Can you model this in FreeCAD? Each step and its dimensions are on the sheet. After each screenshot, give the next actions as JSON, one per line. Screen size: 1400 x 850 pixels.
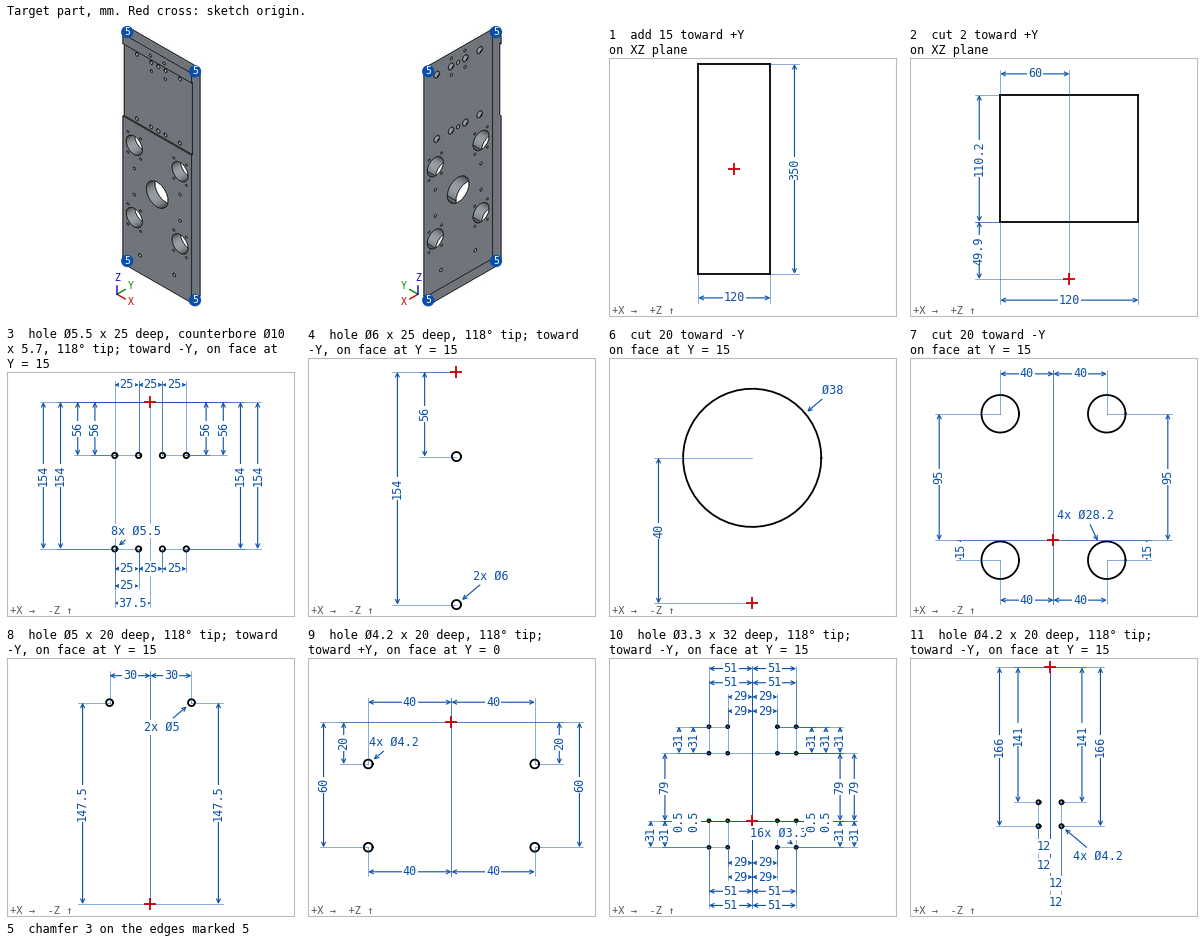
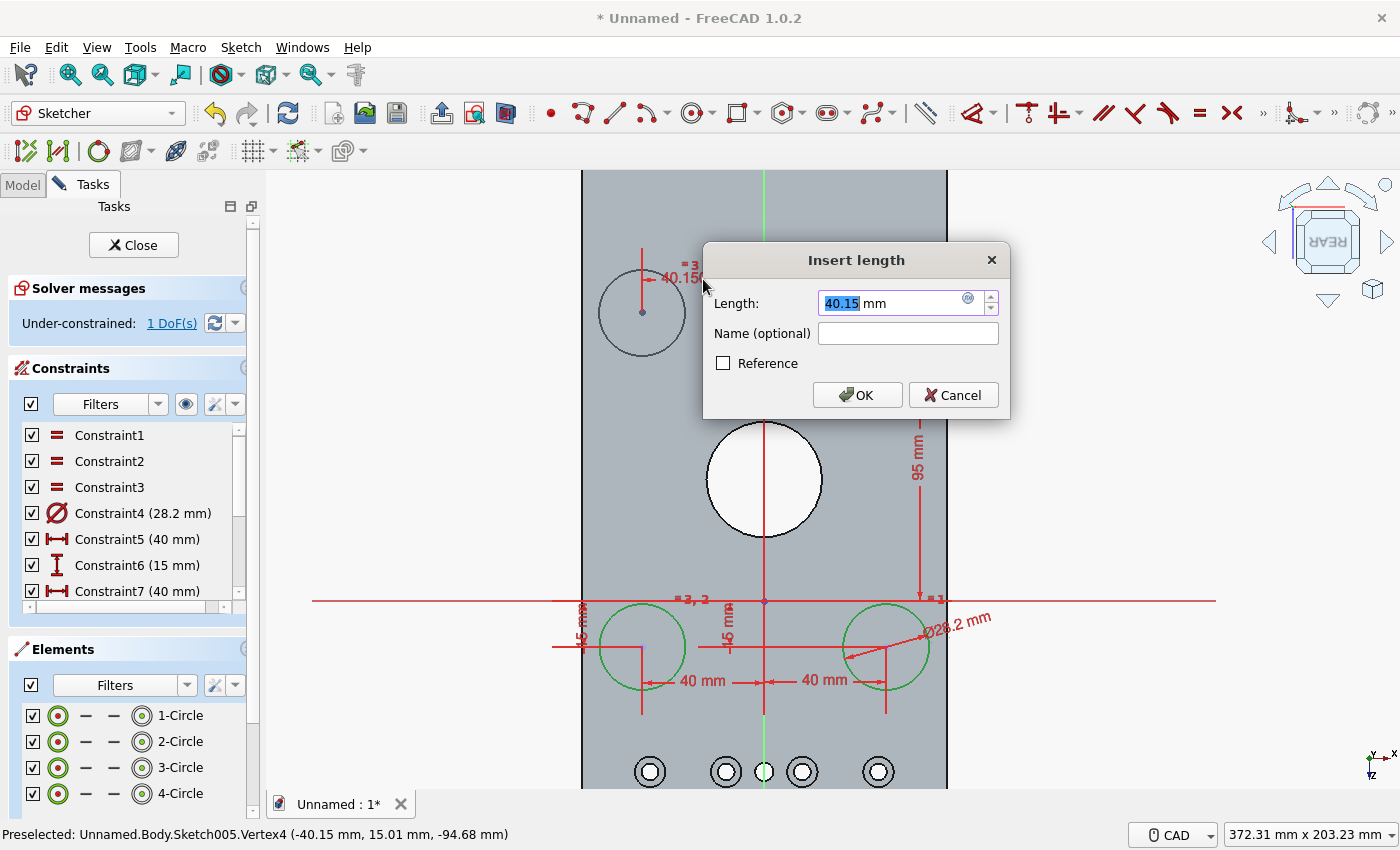
{"action": "type", "text": "40"}
{"action": "key", "text": "Return"}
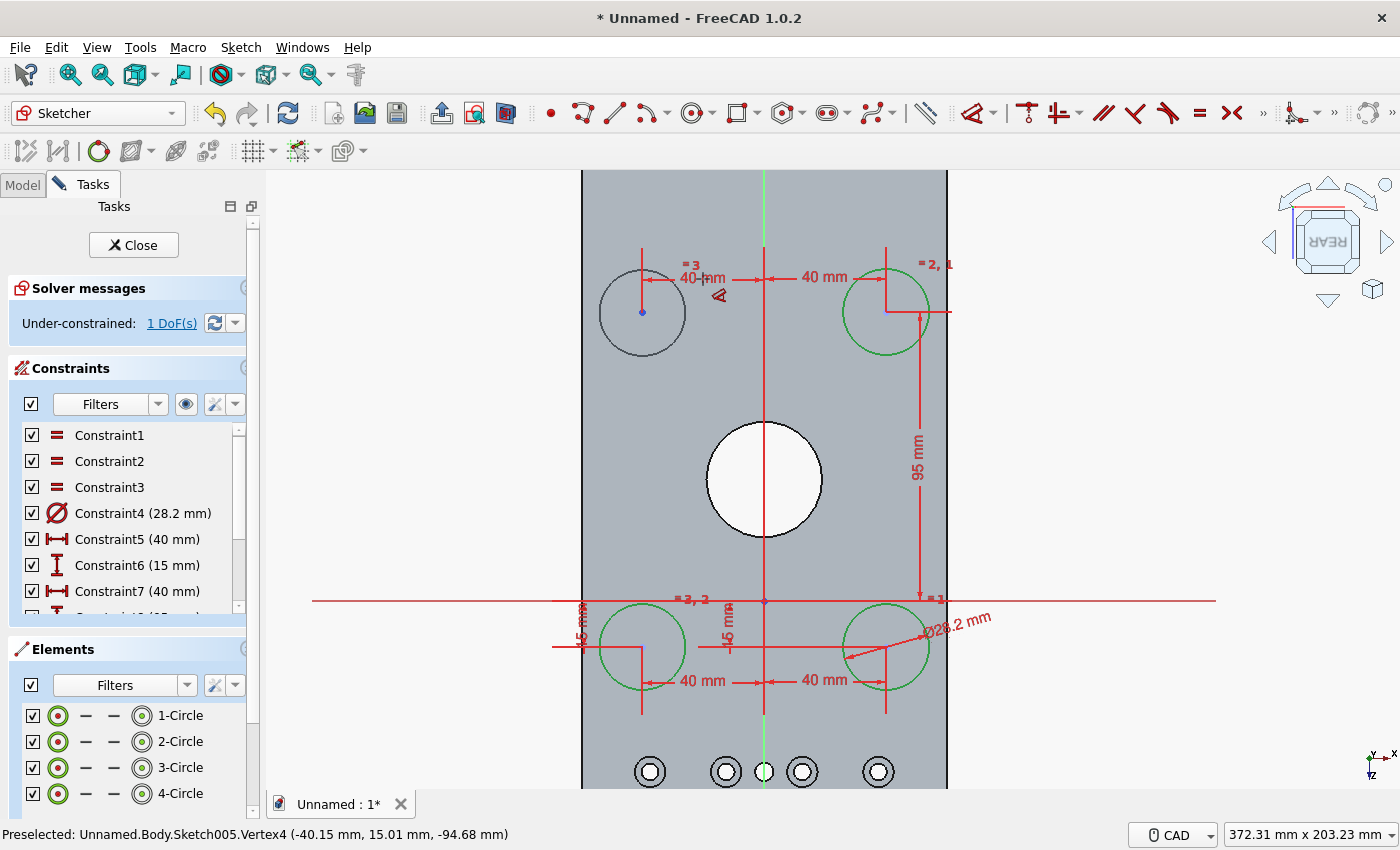
{"action": "left_click", "coordinate": [642, 313]}
{"action": "left_click", "coordinate": [608, 457]}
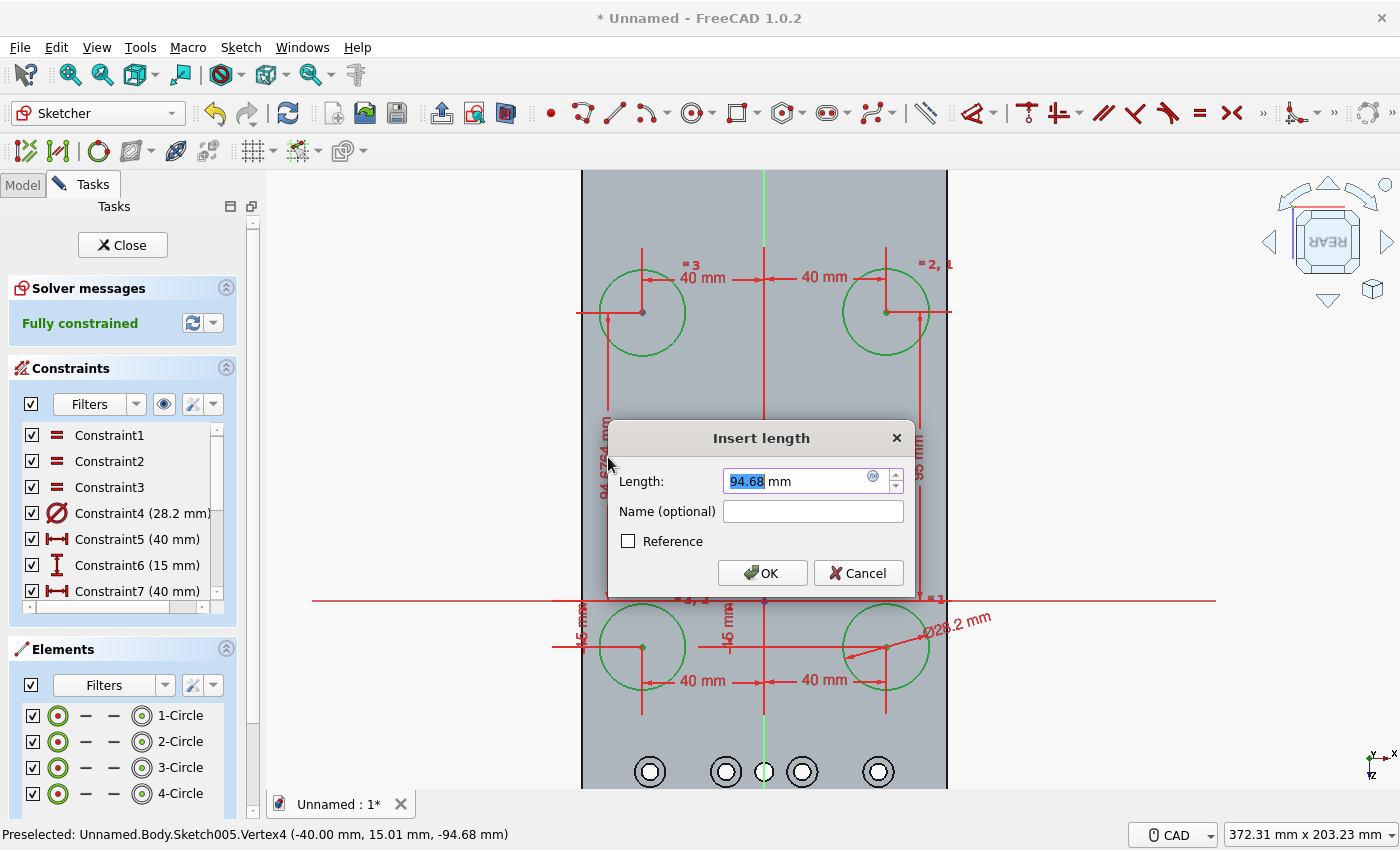
{"action": "type", "text": "95"}
{"action": "key", "text": "Return"}
{"action": "key", "text": "Escape"}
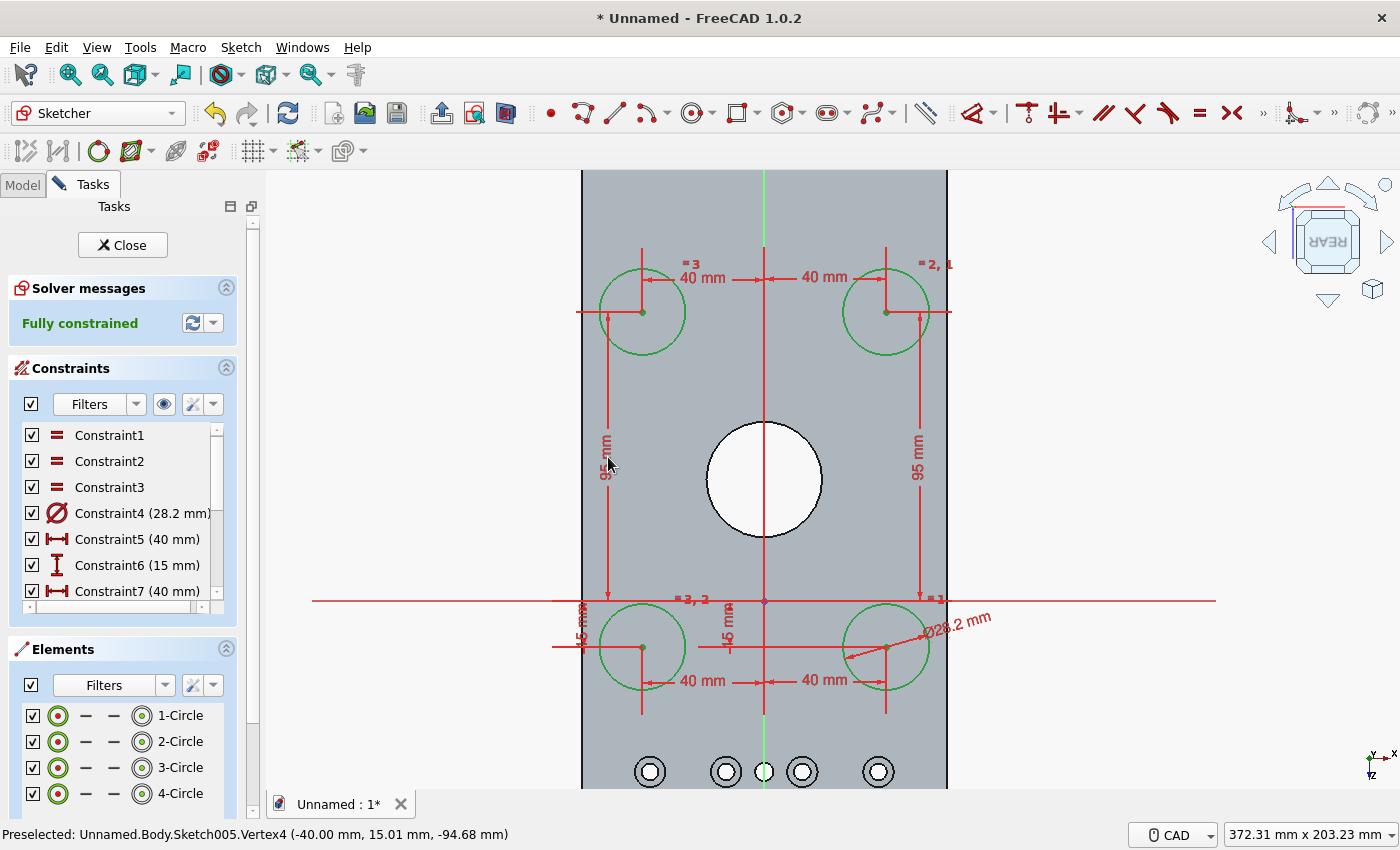
{"action": "left_click", "coordinate": [123, 245]}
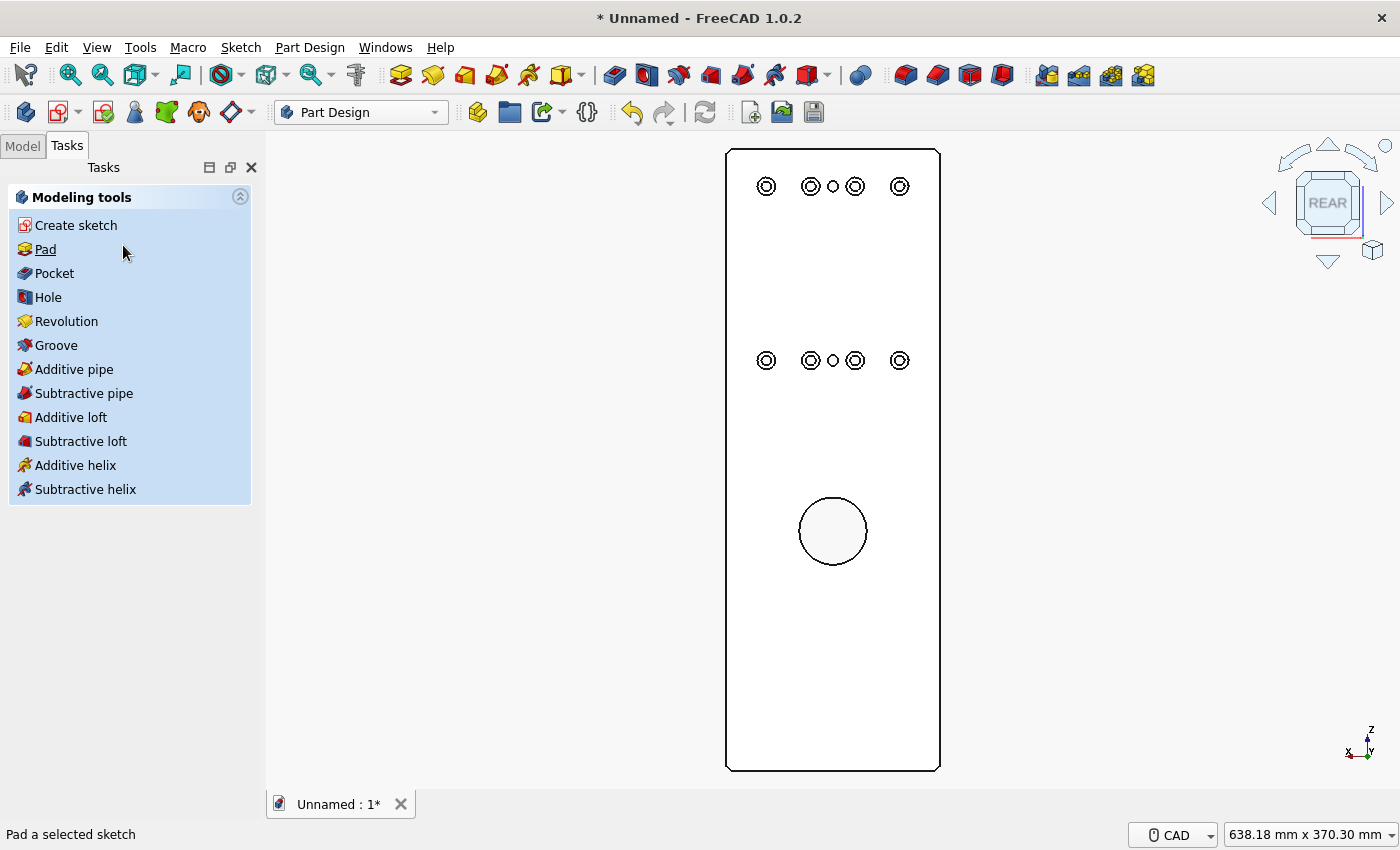
{"action": "left_click", "coordinate": [616, 76]}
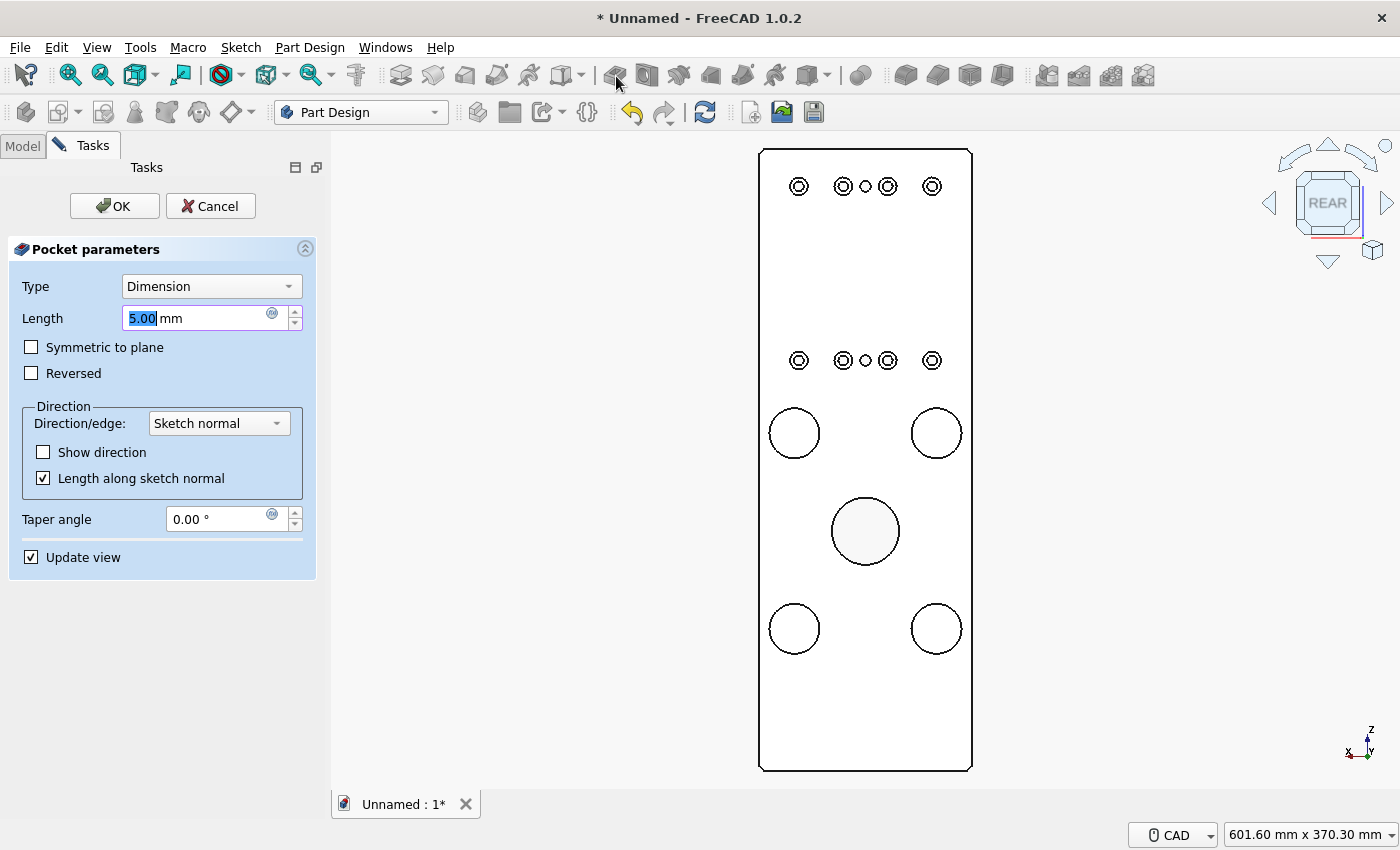
{"action": "type", "text": "20"}
{"action": "key", "text": "Tab"}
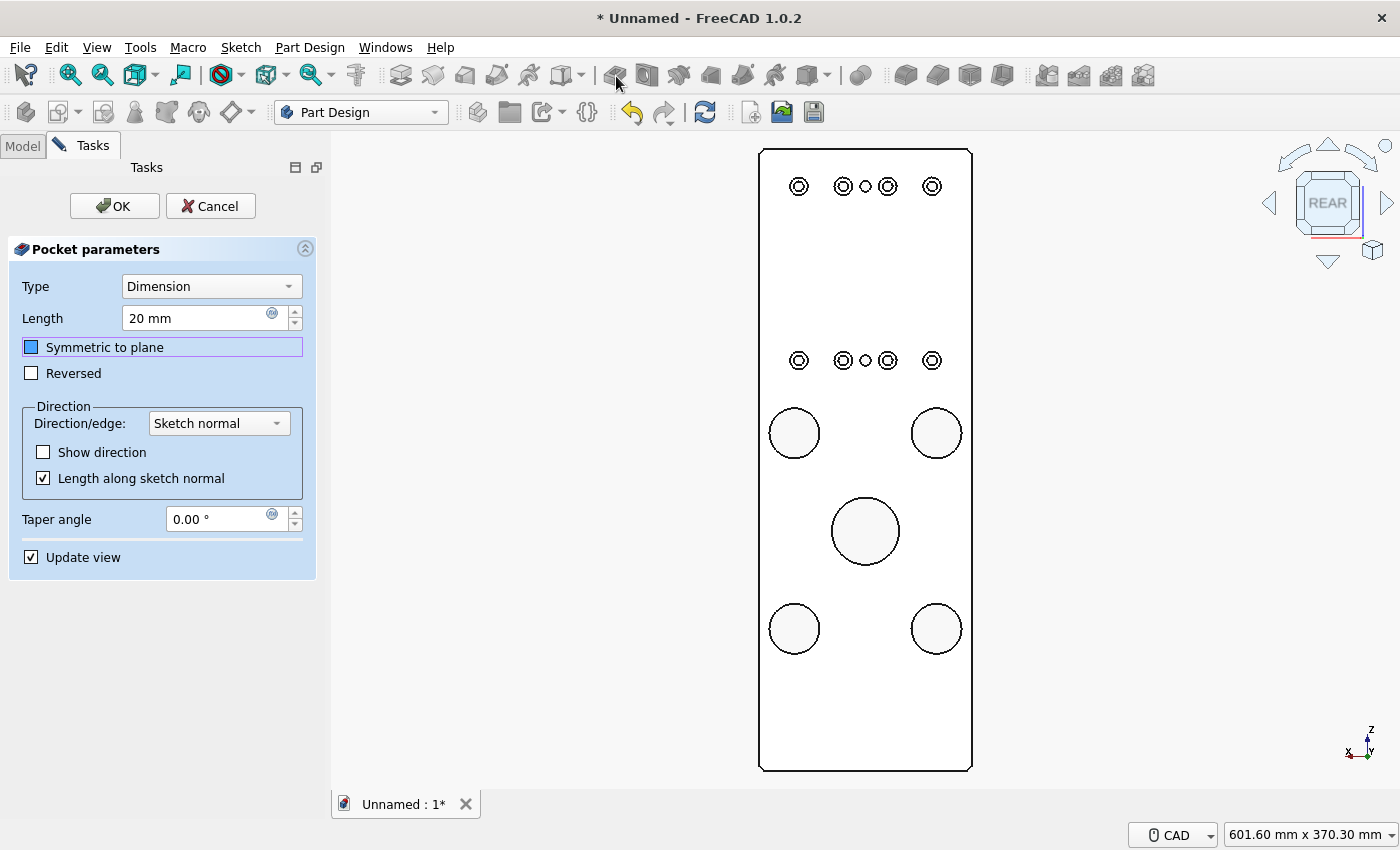
{"action": "left_click", "coordinate": [115, 206]}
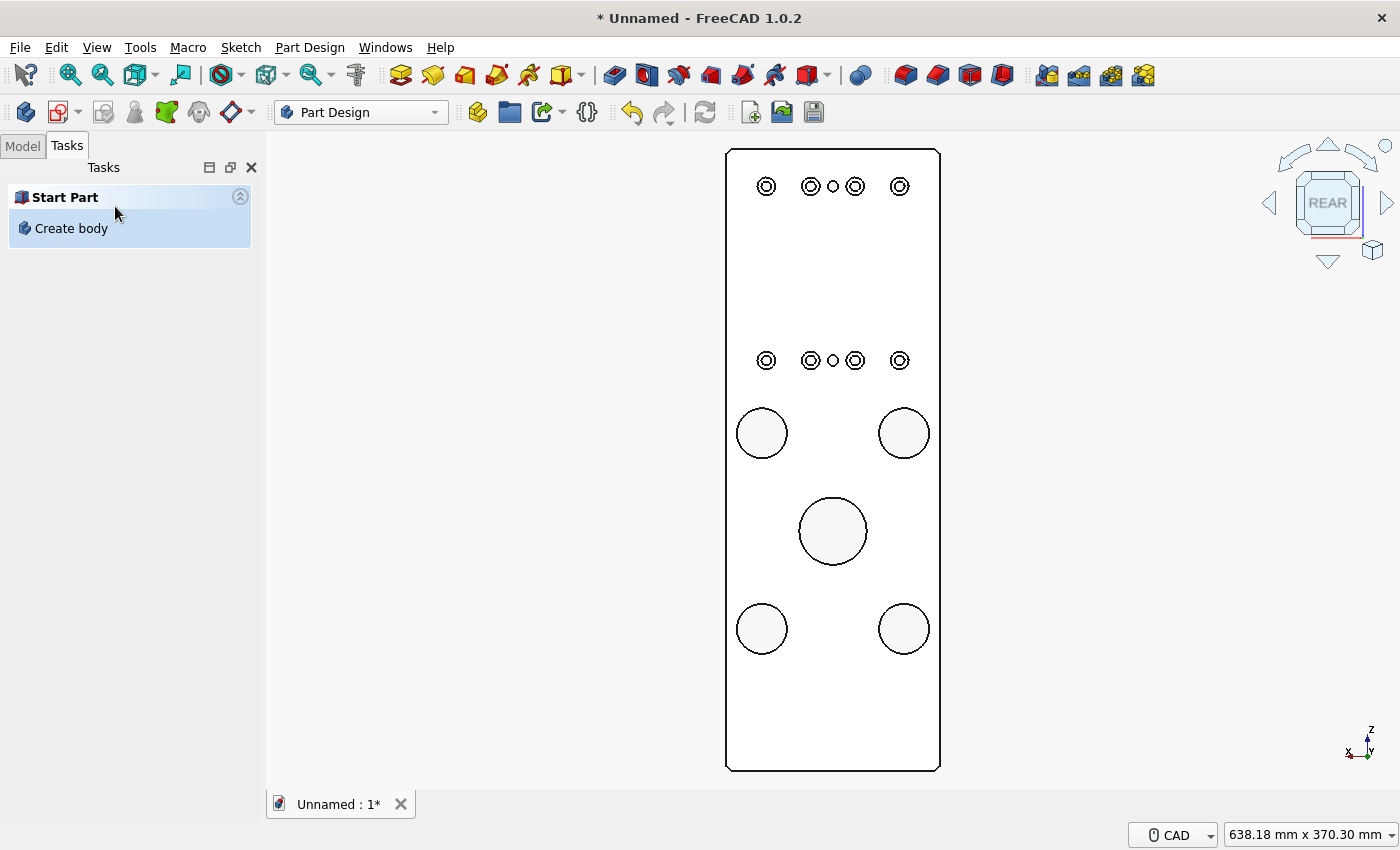
{"action": "left_click", "coordinate": [833, 281]}